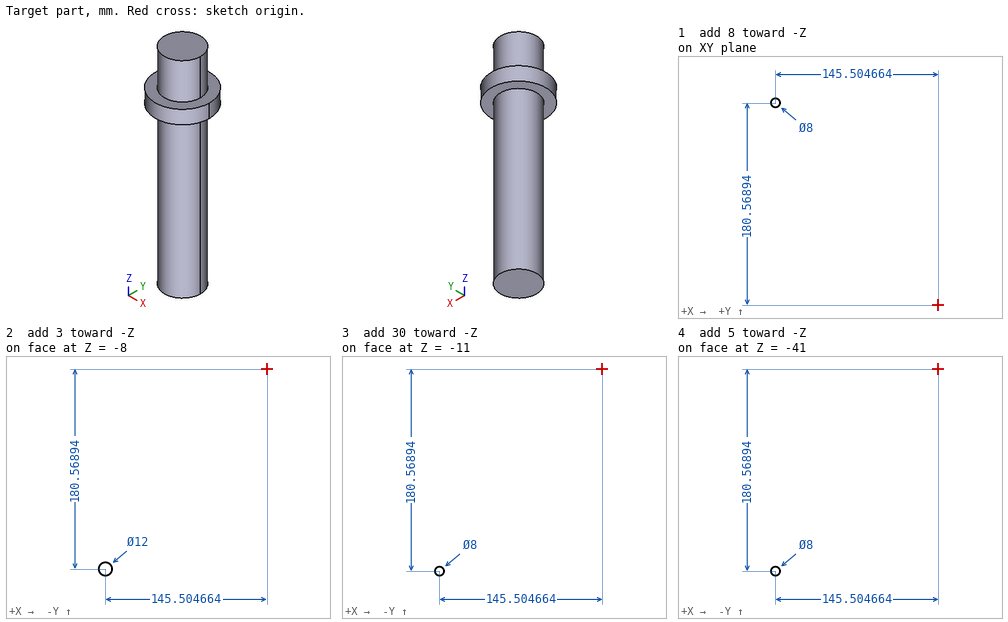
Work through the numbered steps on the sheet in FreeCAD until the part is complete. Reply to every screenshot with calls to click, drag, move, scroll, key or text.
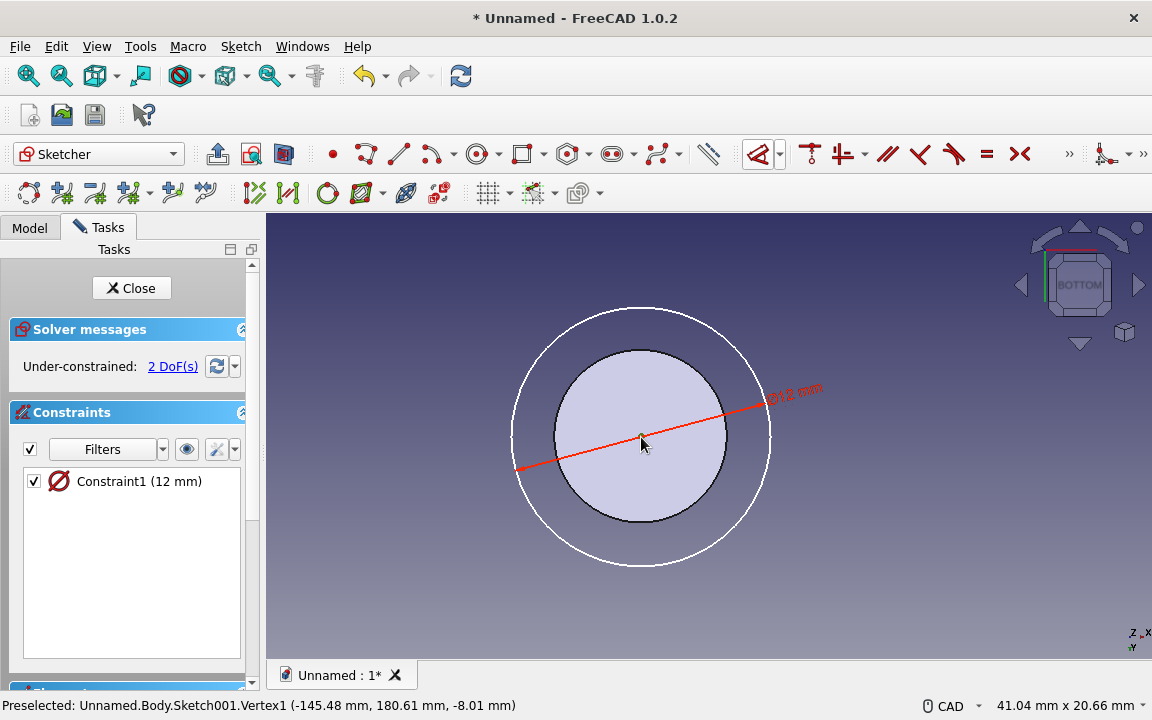
click(780, 154)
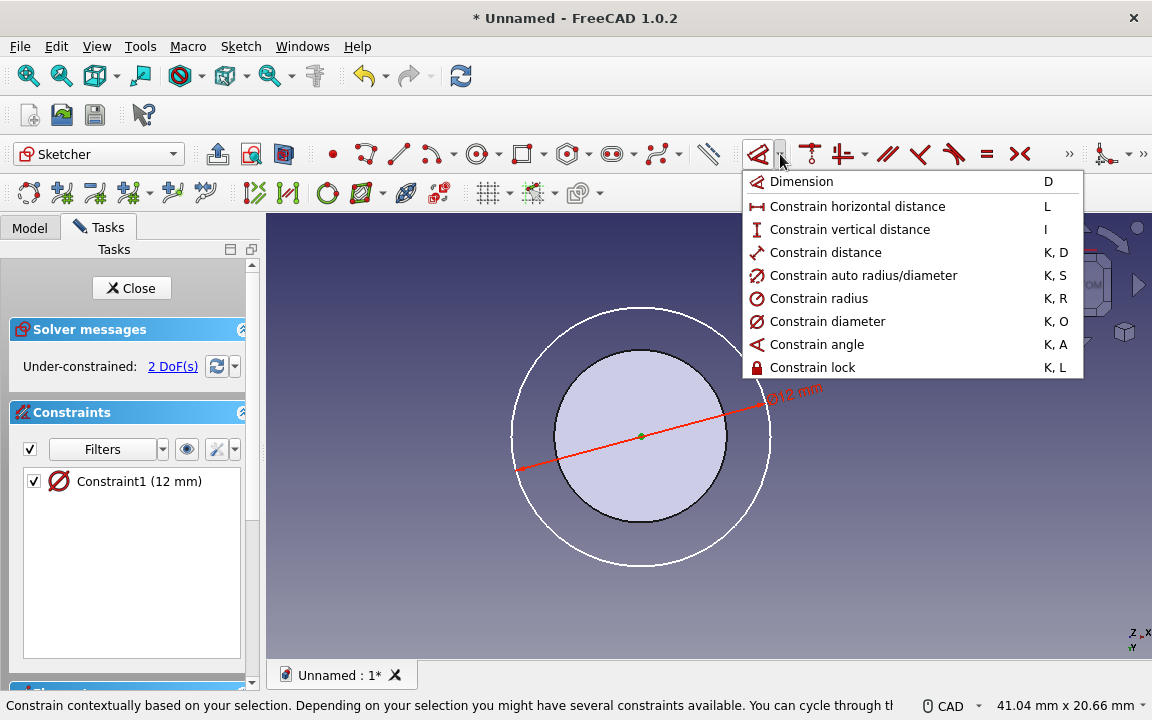
click(913, 230)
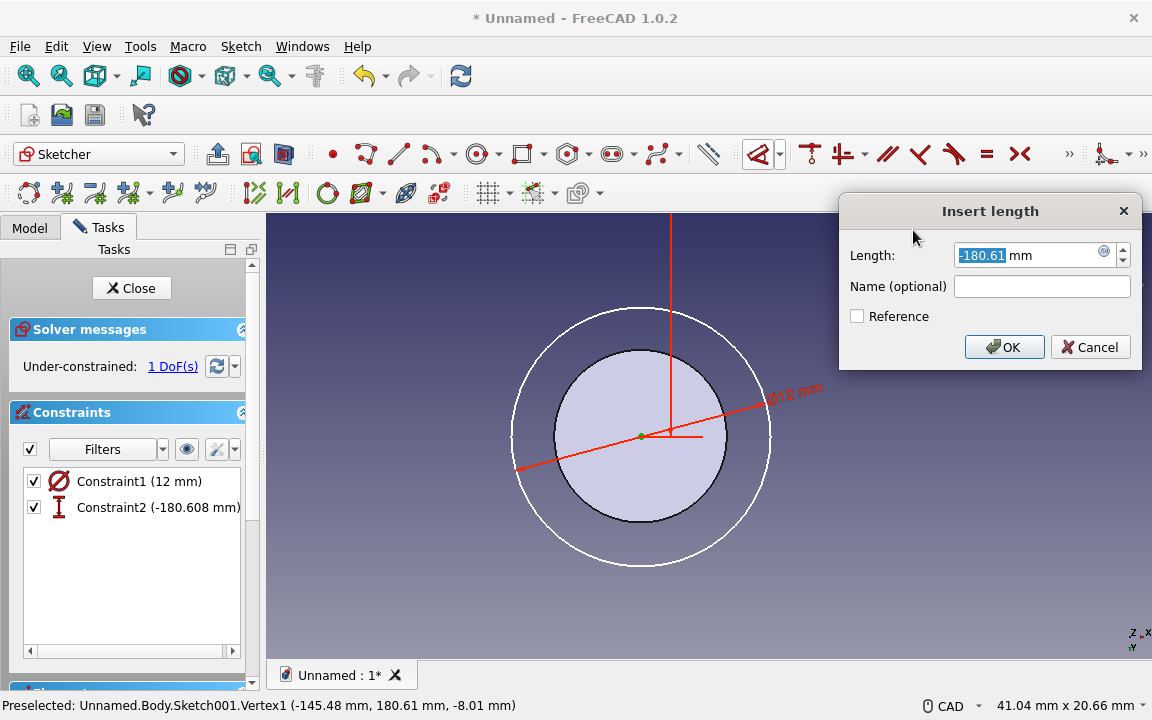
text(-180.56894)
key(Return)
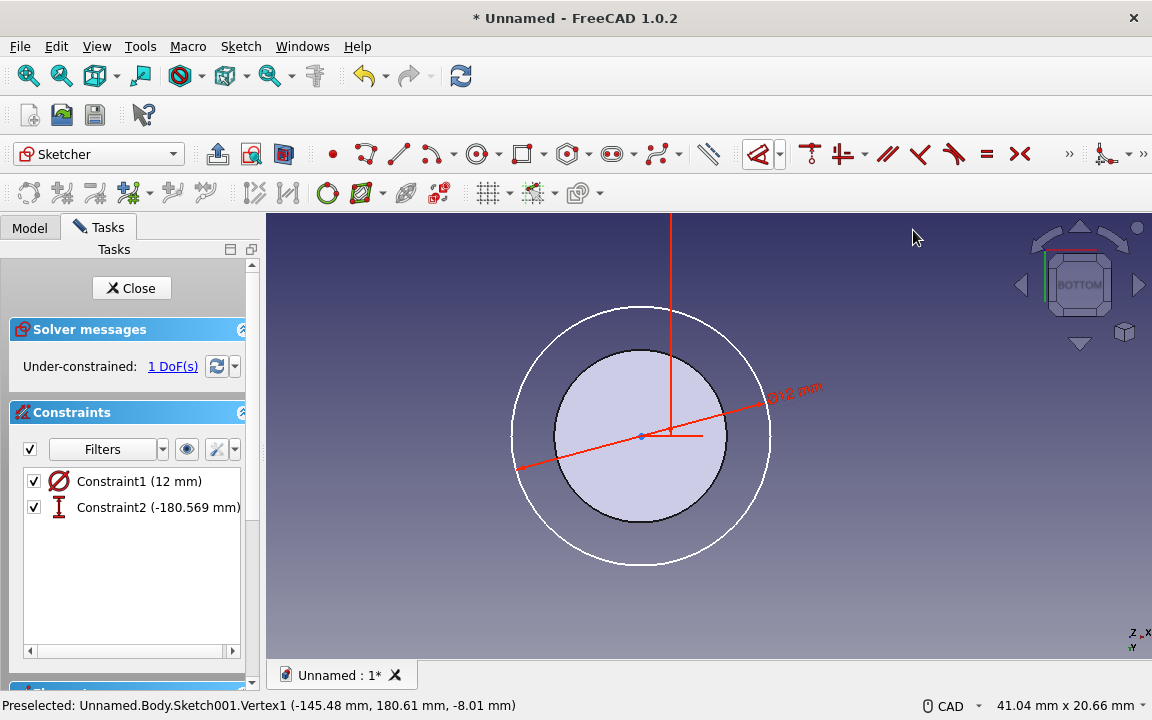
click(641, 436)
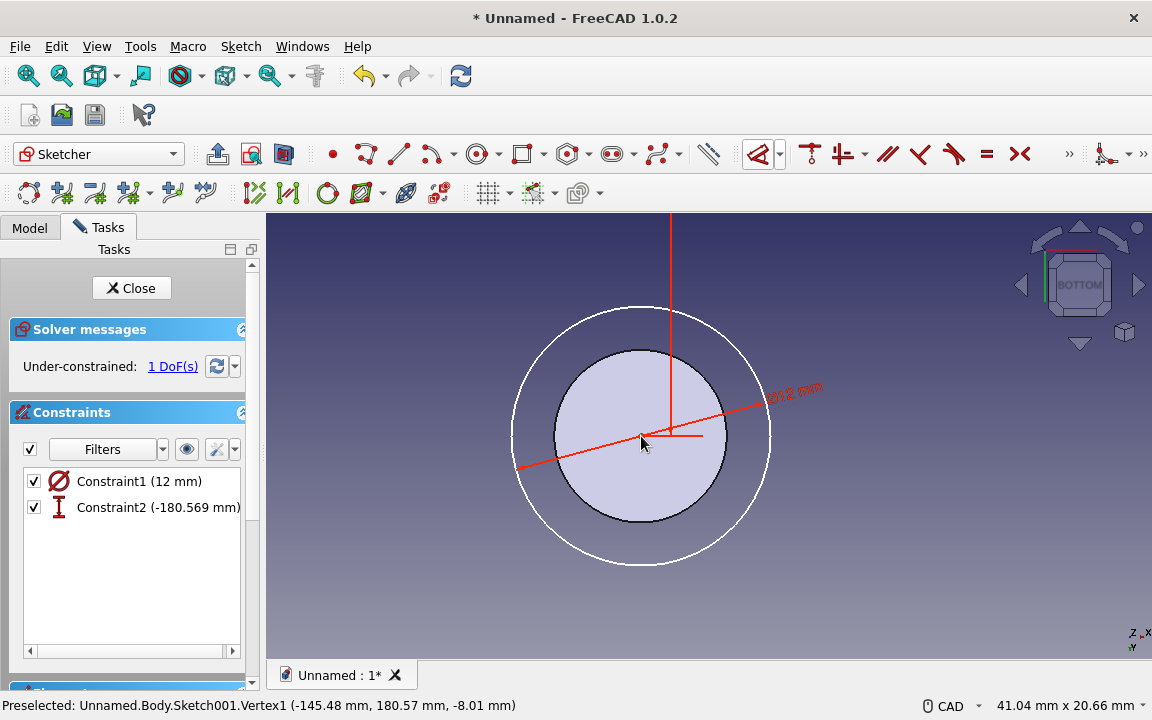
key(l)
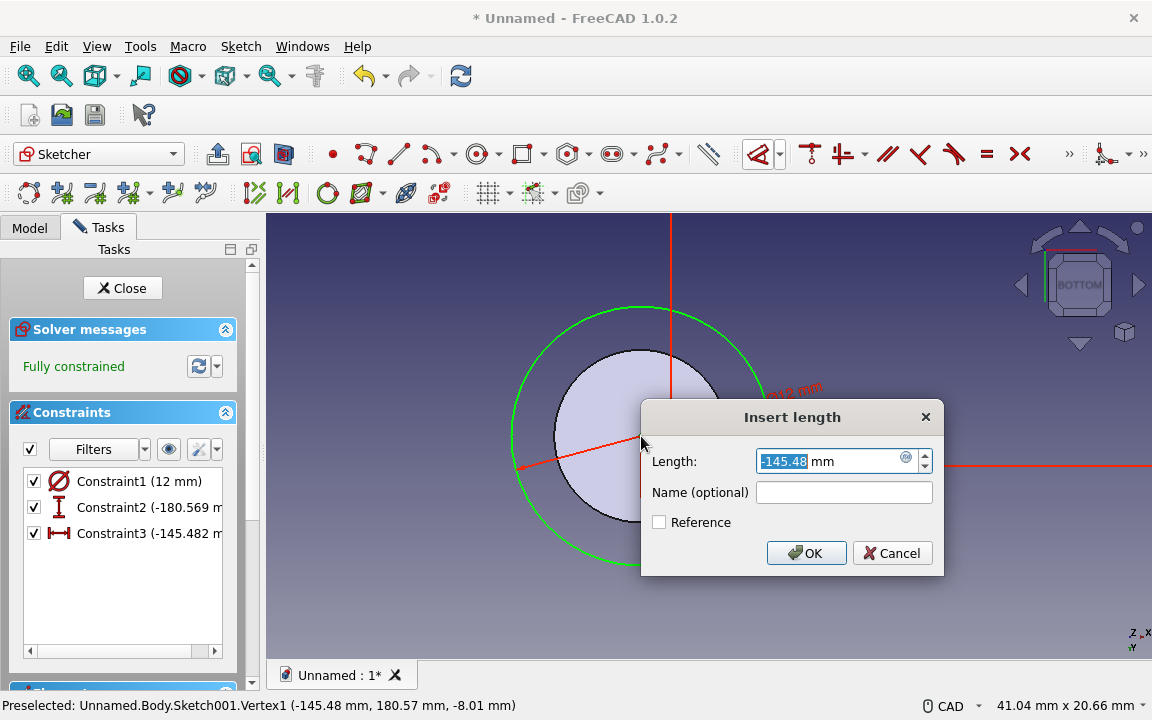
text(-145.504664)
key(Return)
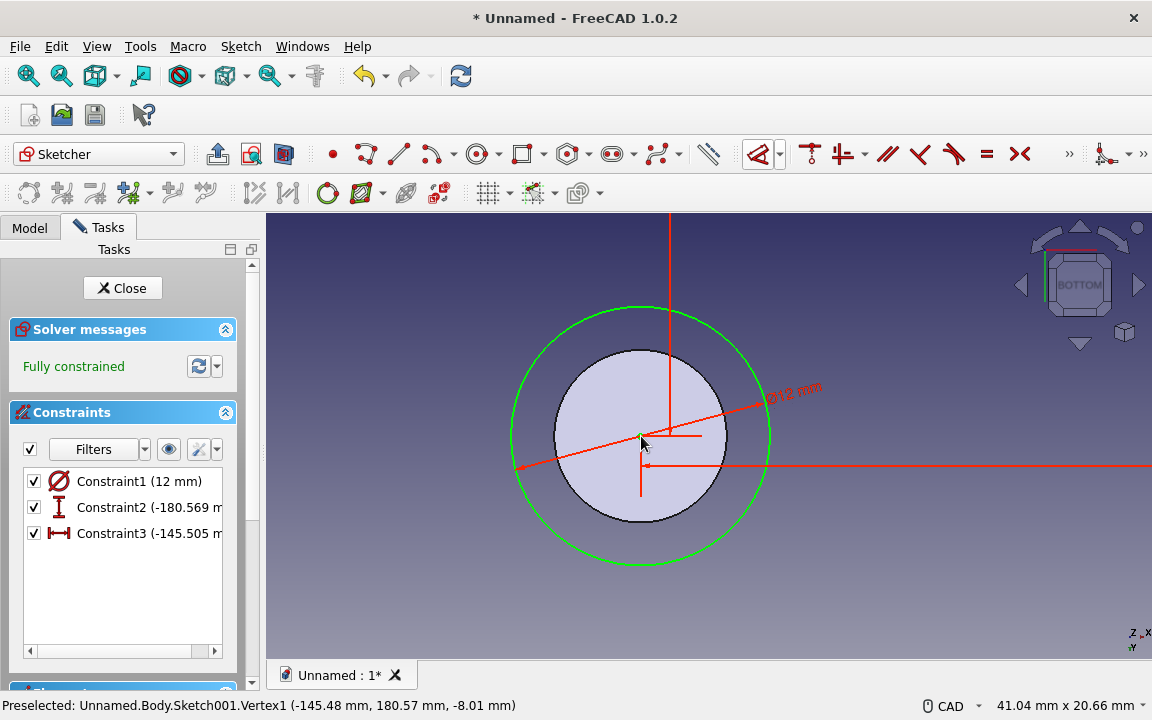
click(123, 288)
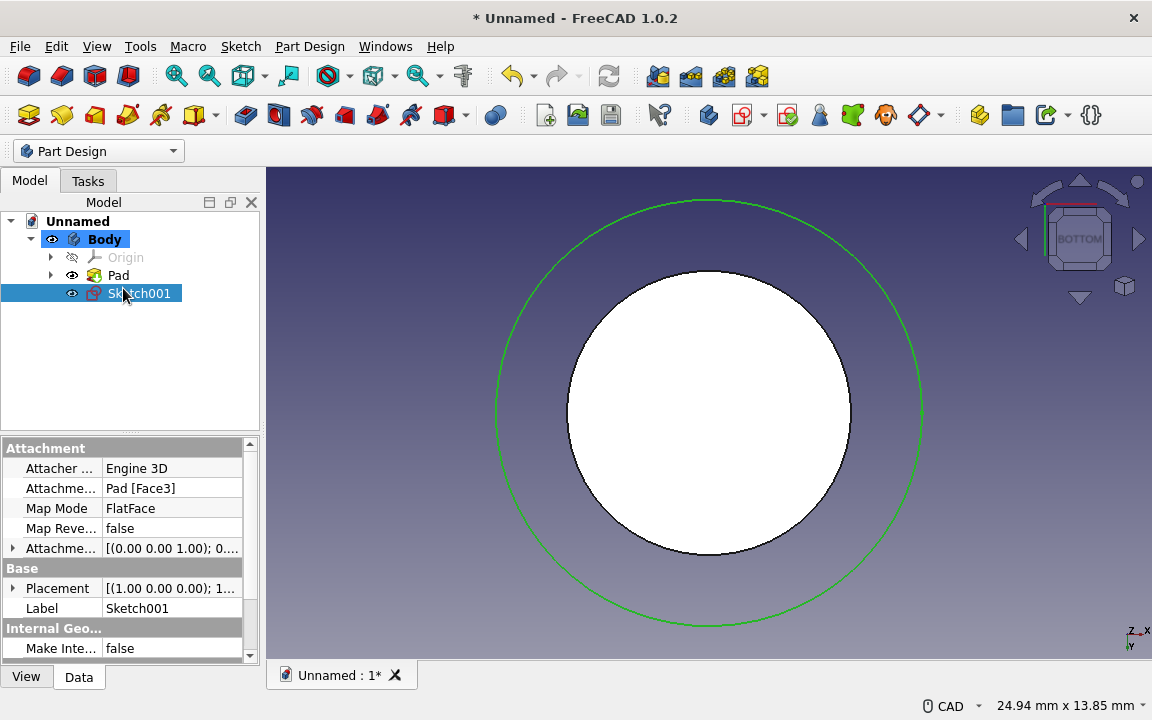
click(29, 116)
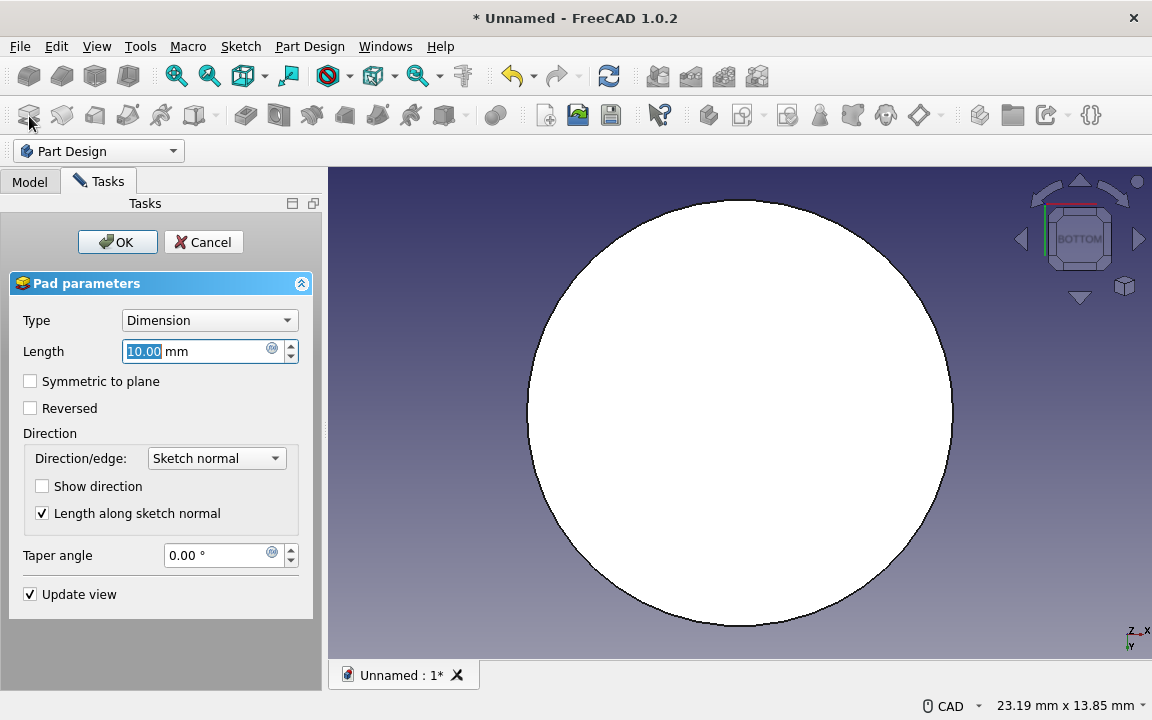
text(3)
key(Tab)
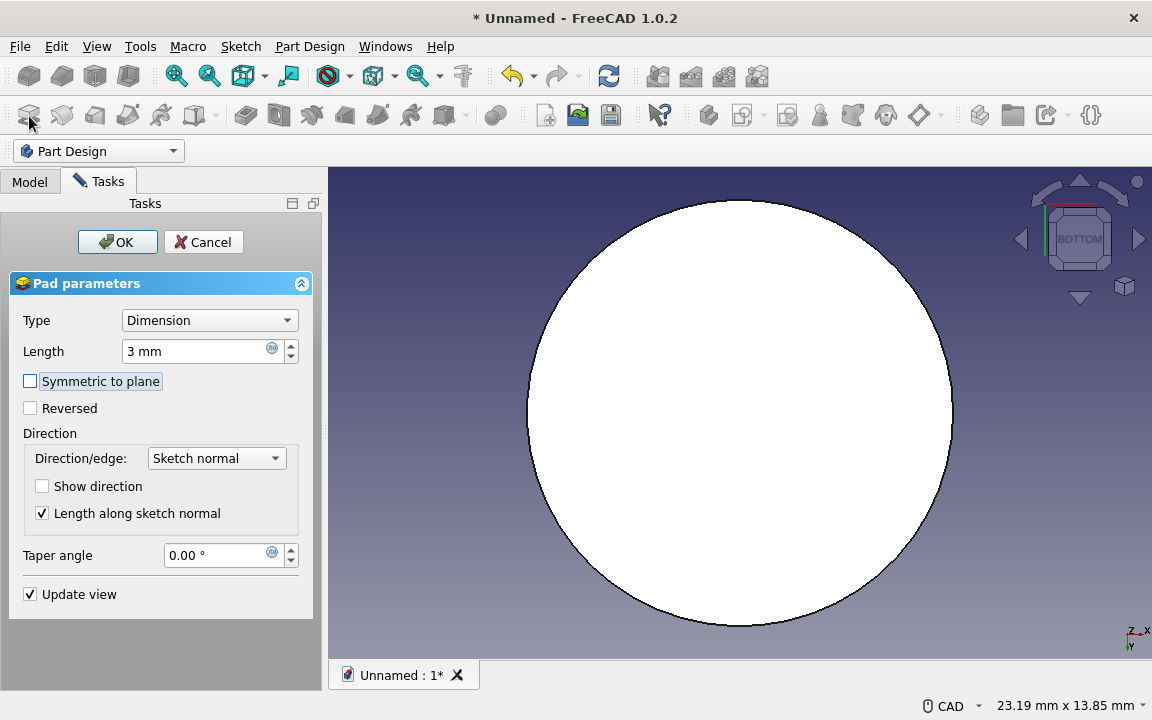
click(118, 242)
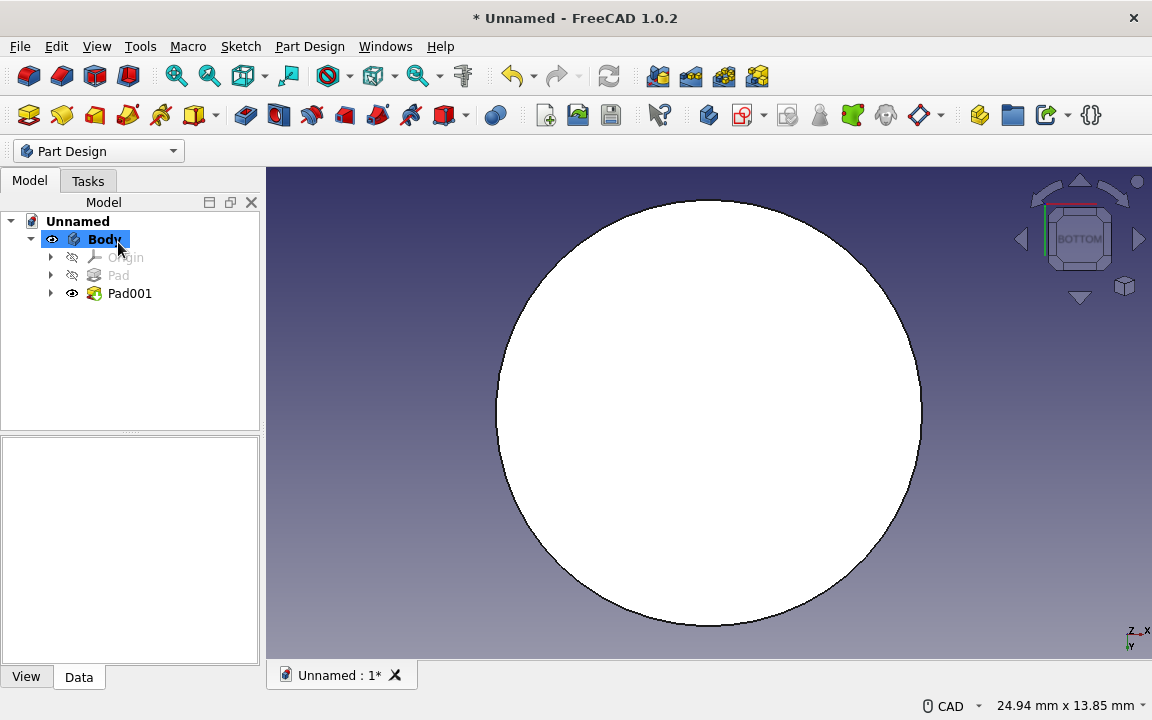
click(709, 412)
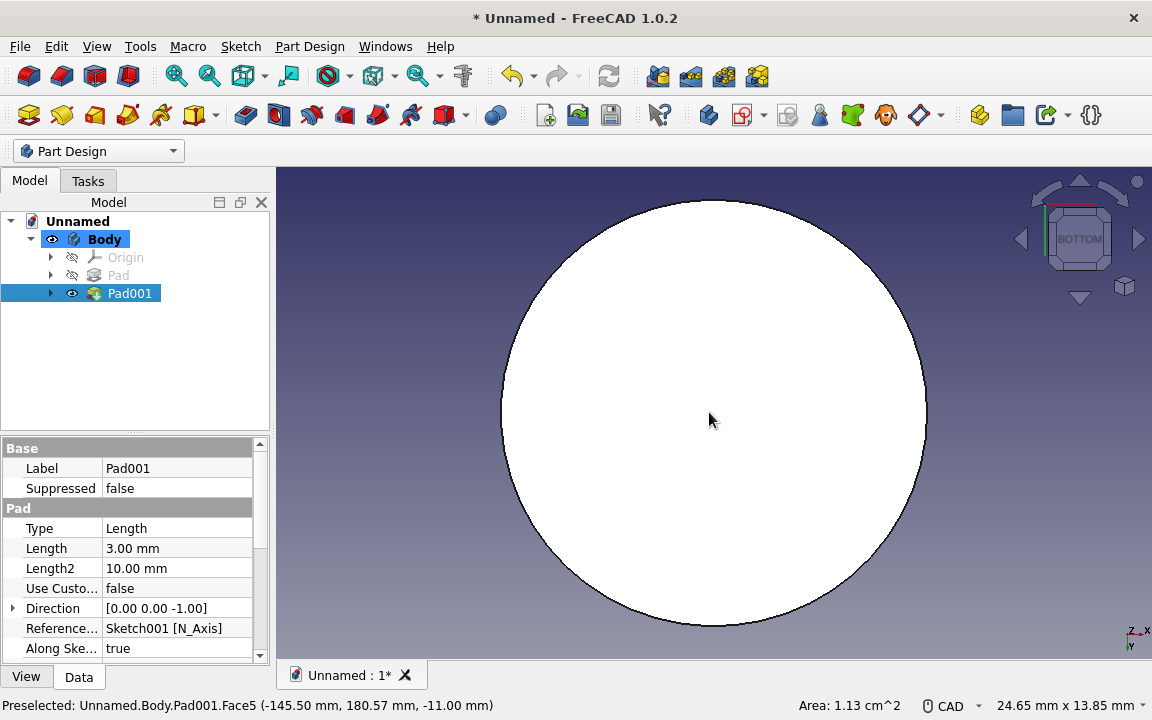
click(742, 116)